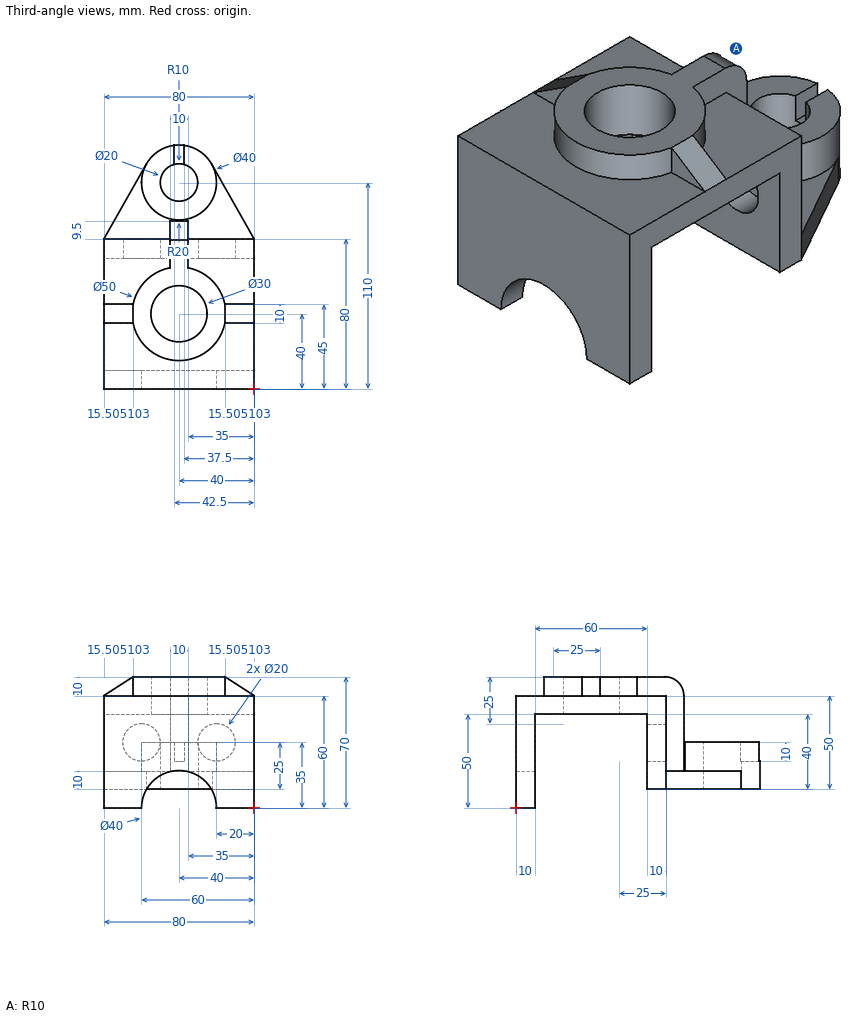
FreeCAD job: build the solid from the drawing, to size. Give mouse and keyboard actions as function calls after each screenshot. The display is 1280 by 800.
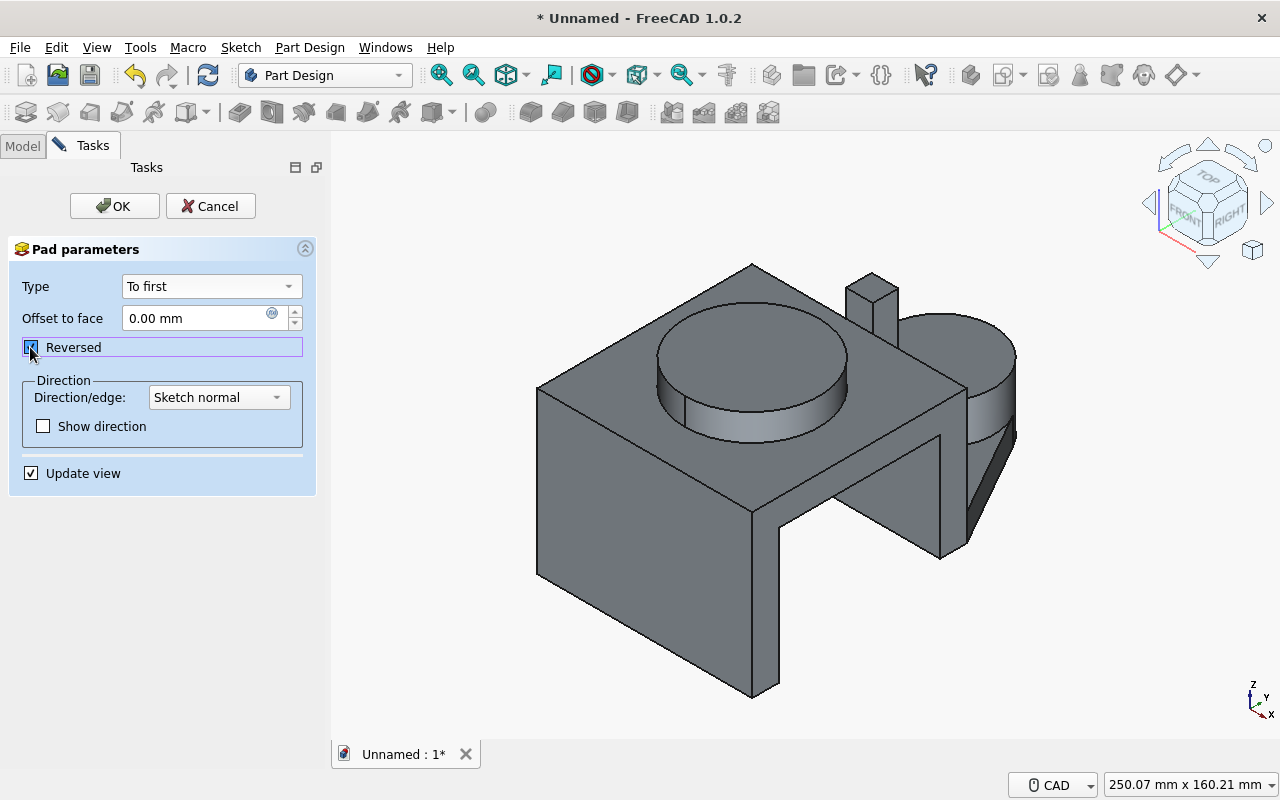
click(115, 206)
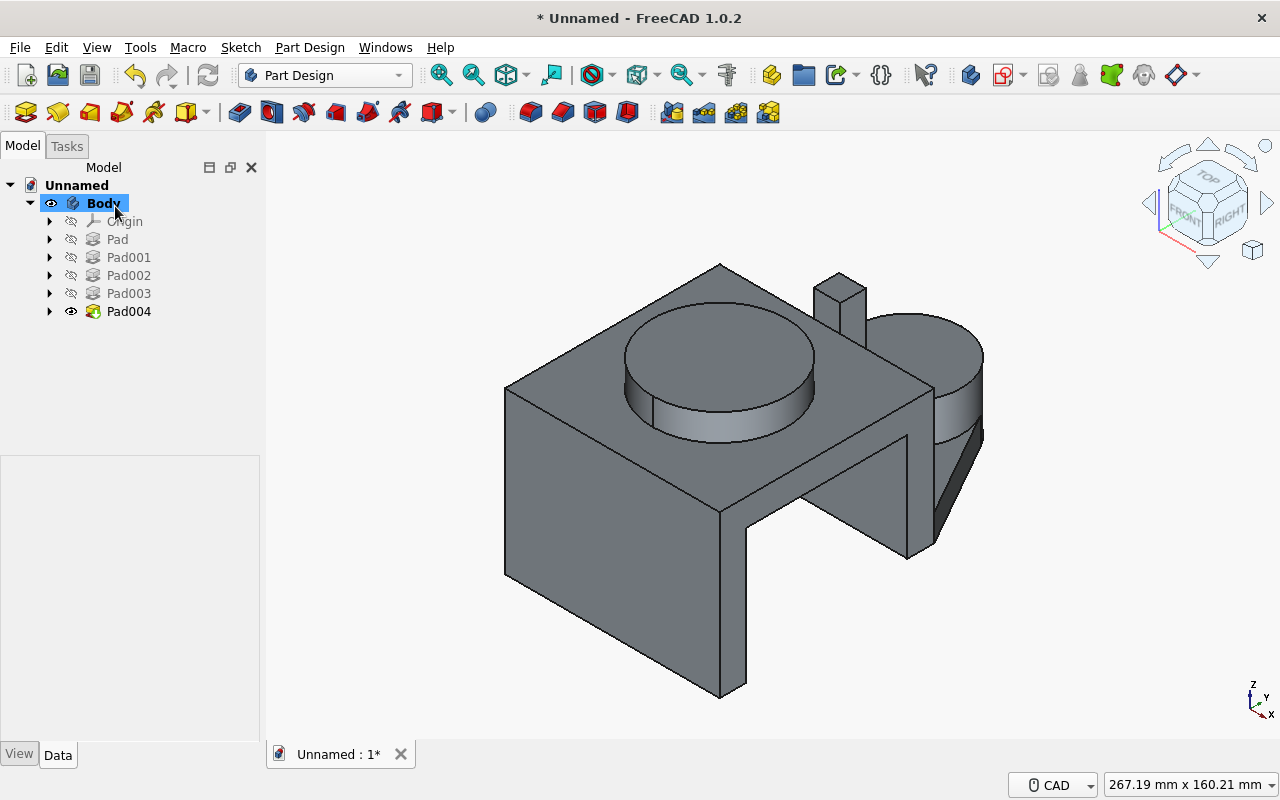
key(4)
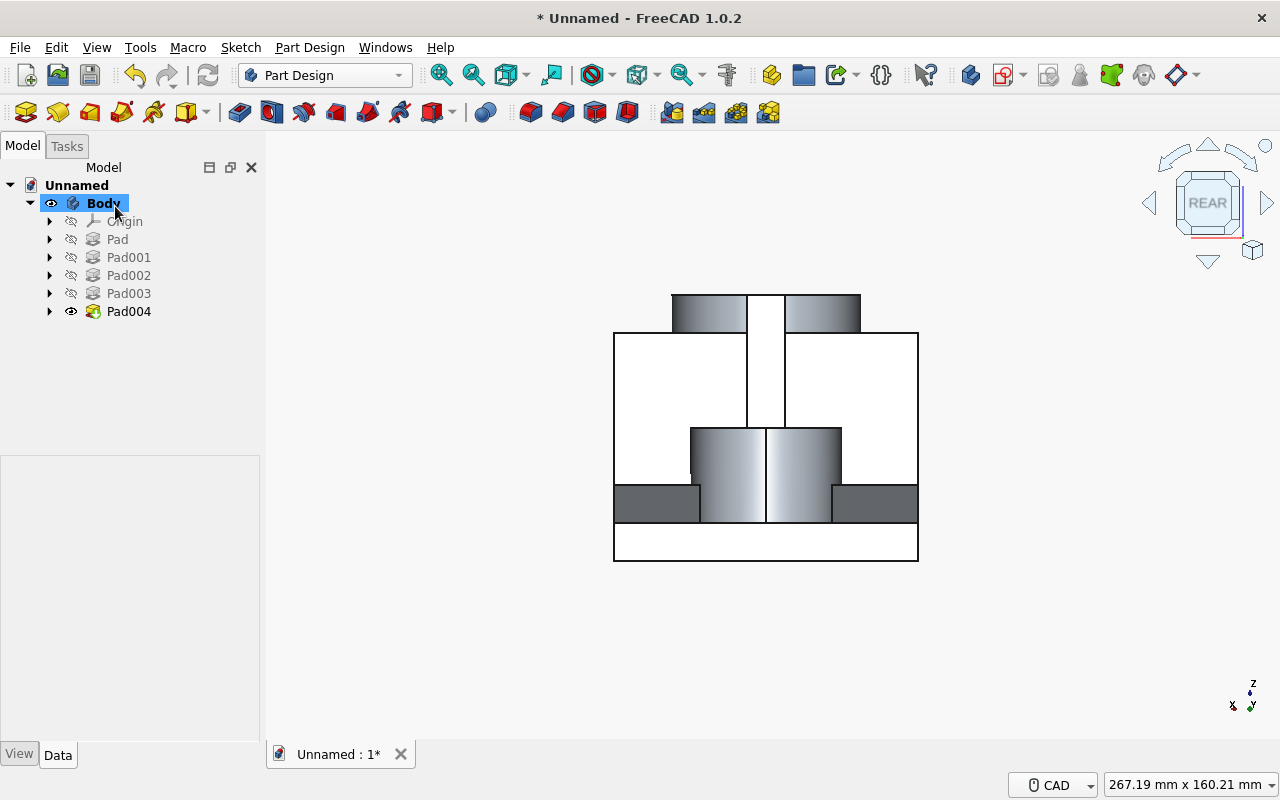
click(442, 76)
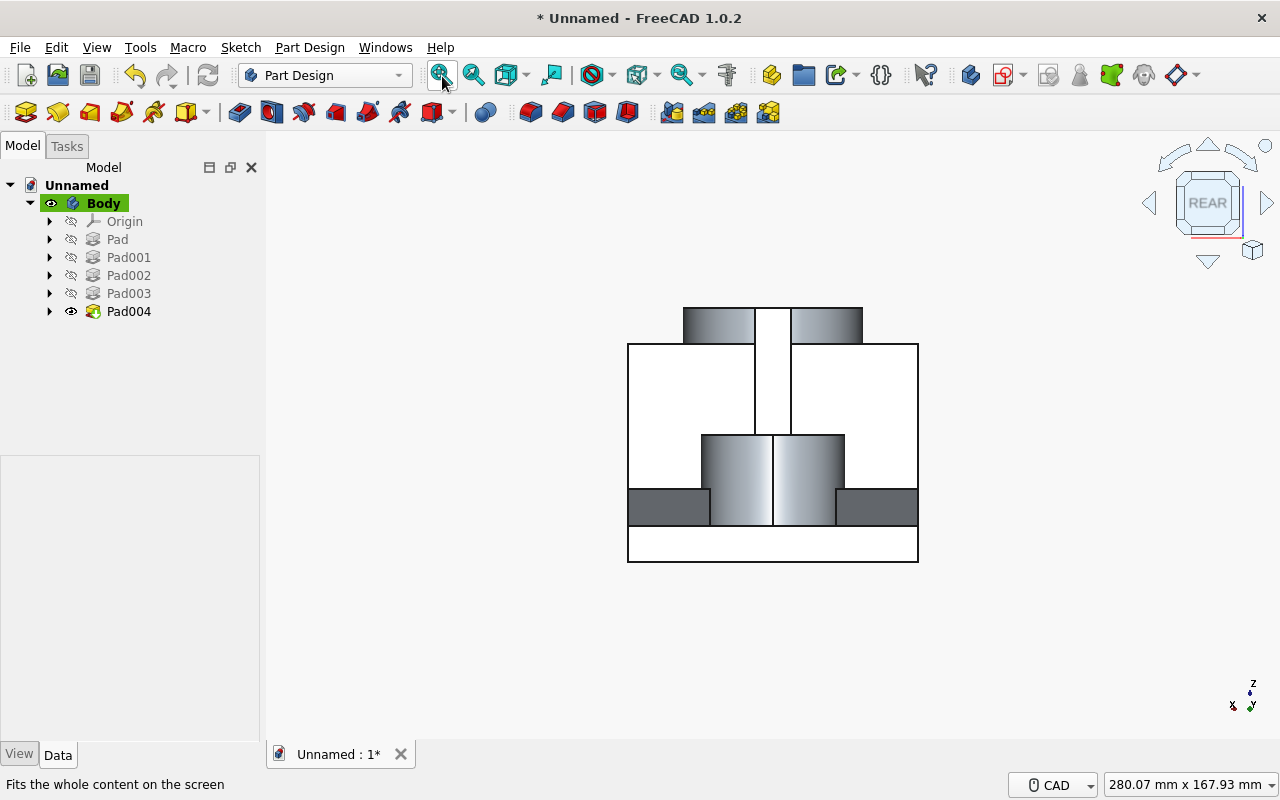
click(692, 416)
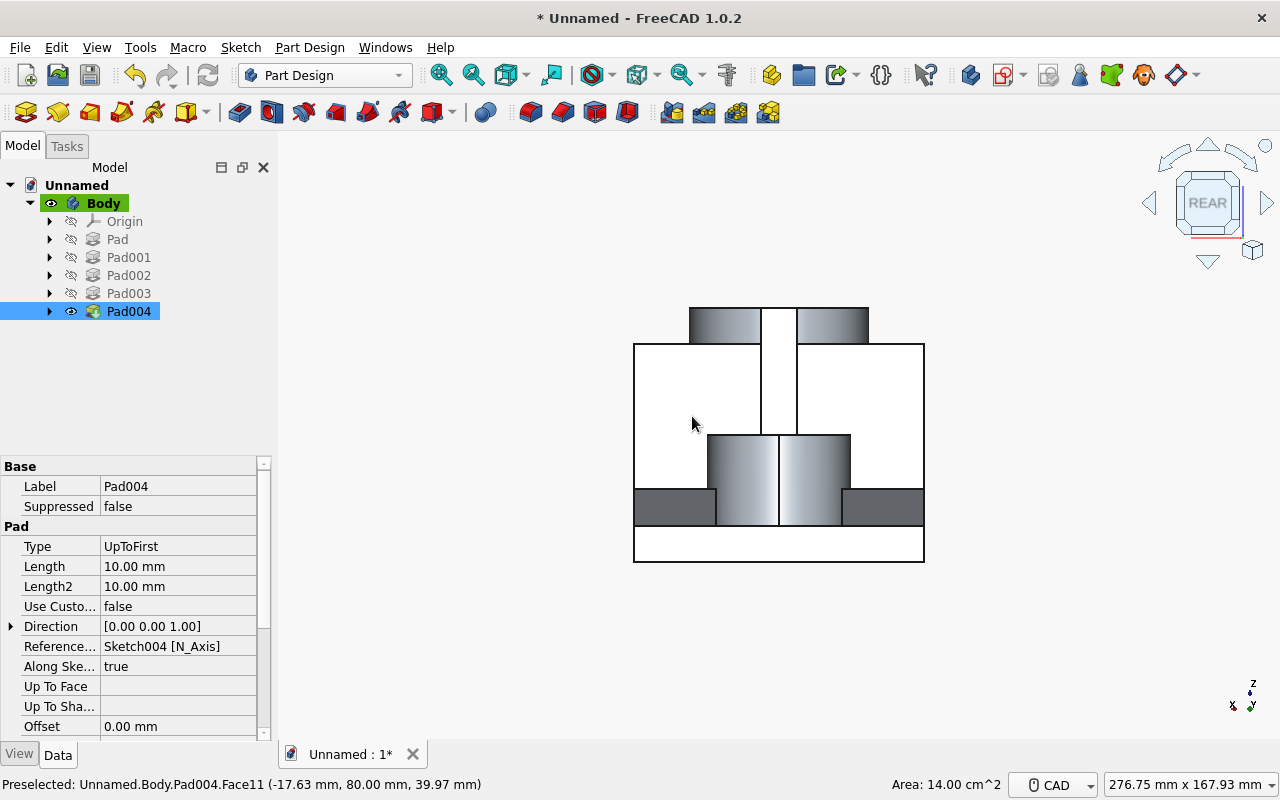
click(1004, 76)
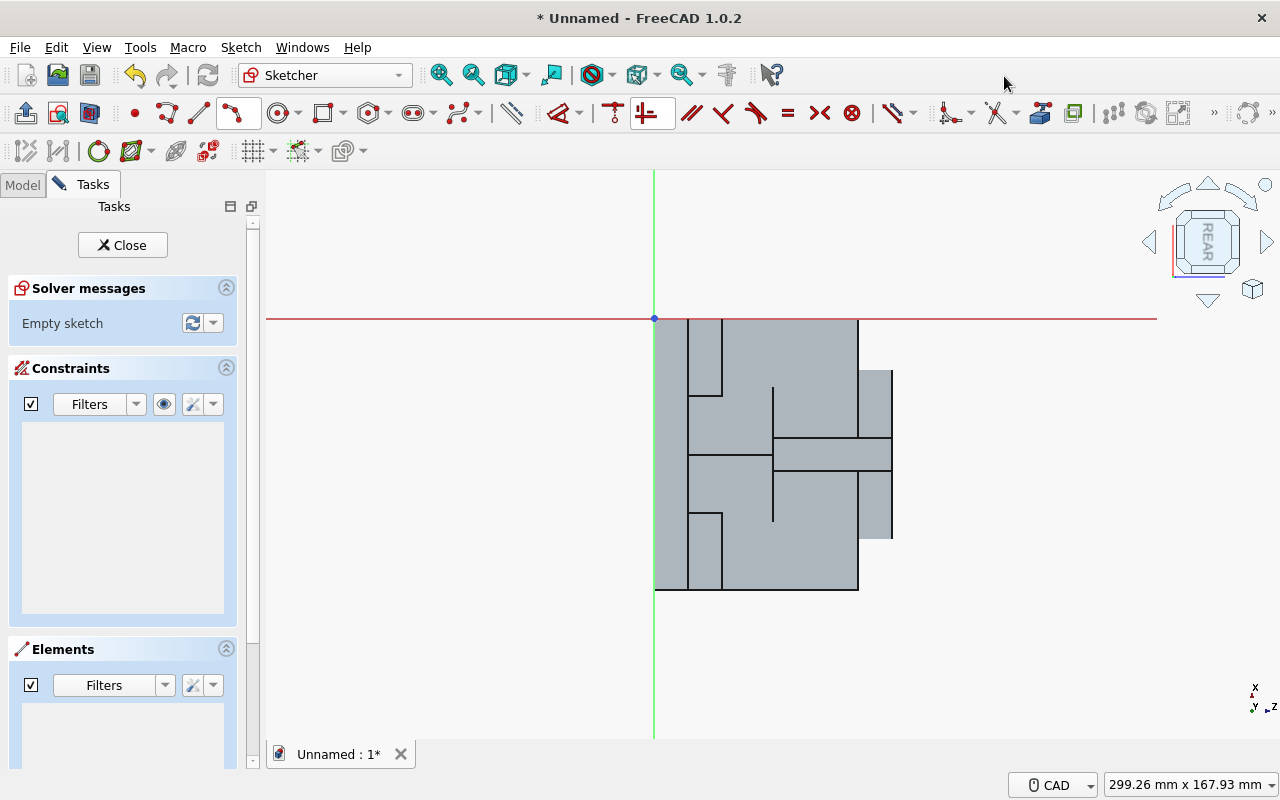
scroll(892, 455, up, 12)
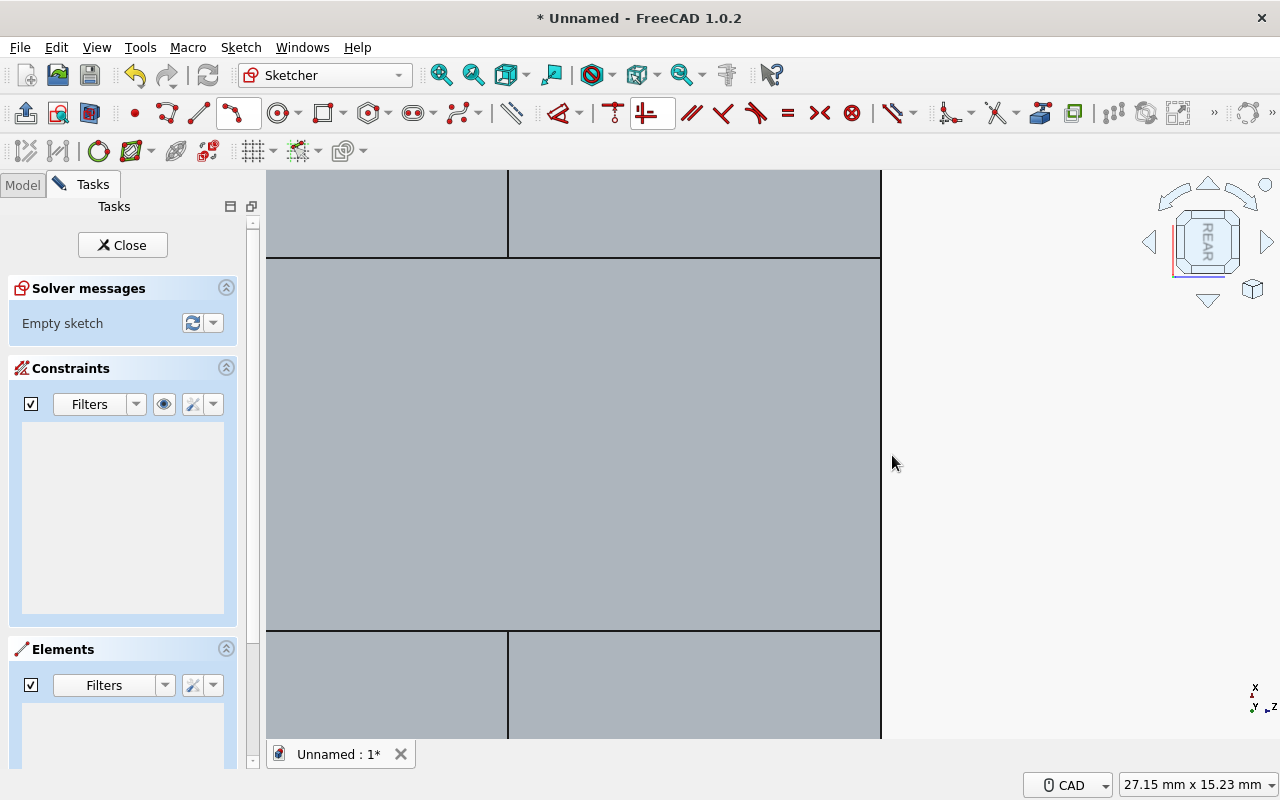
click(324, 114)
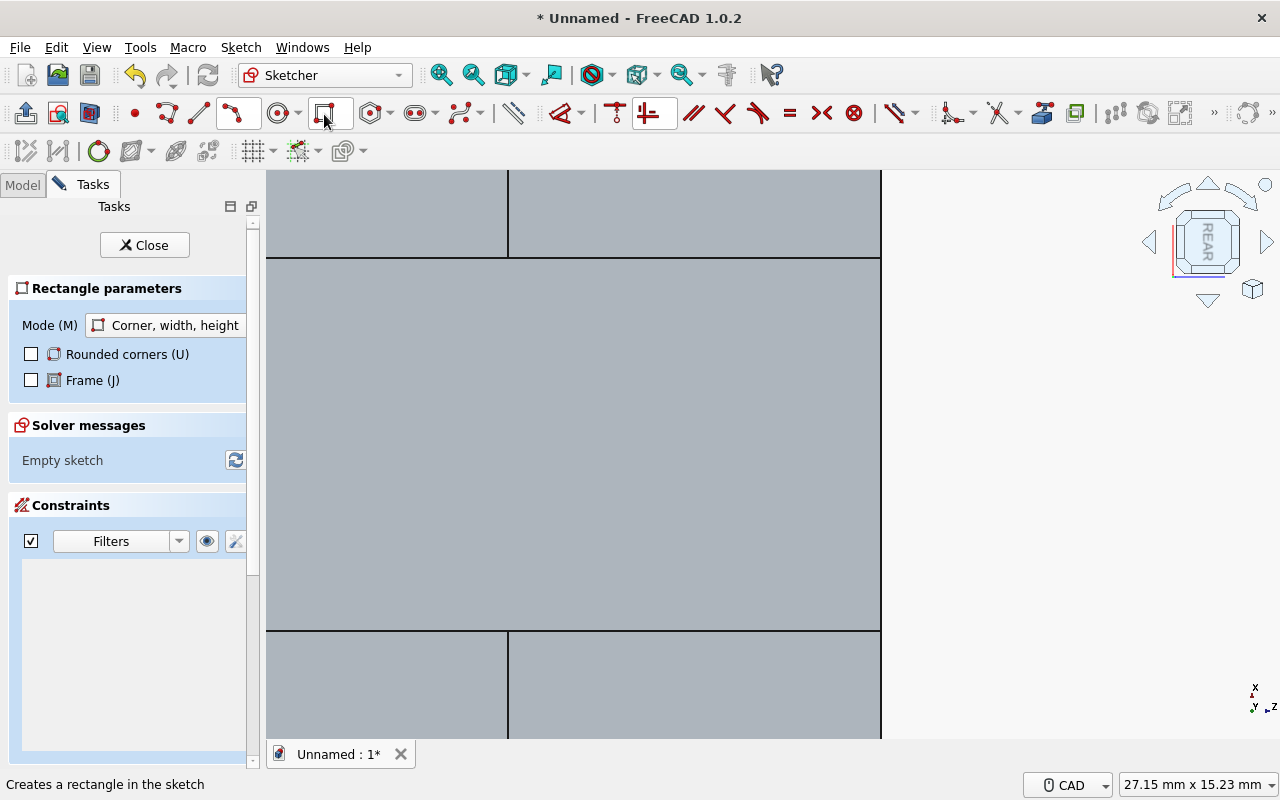
click(508, 258)
move(881, 631)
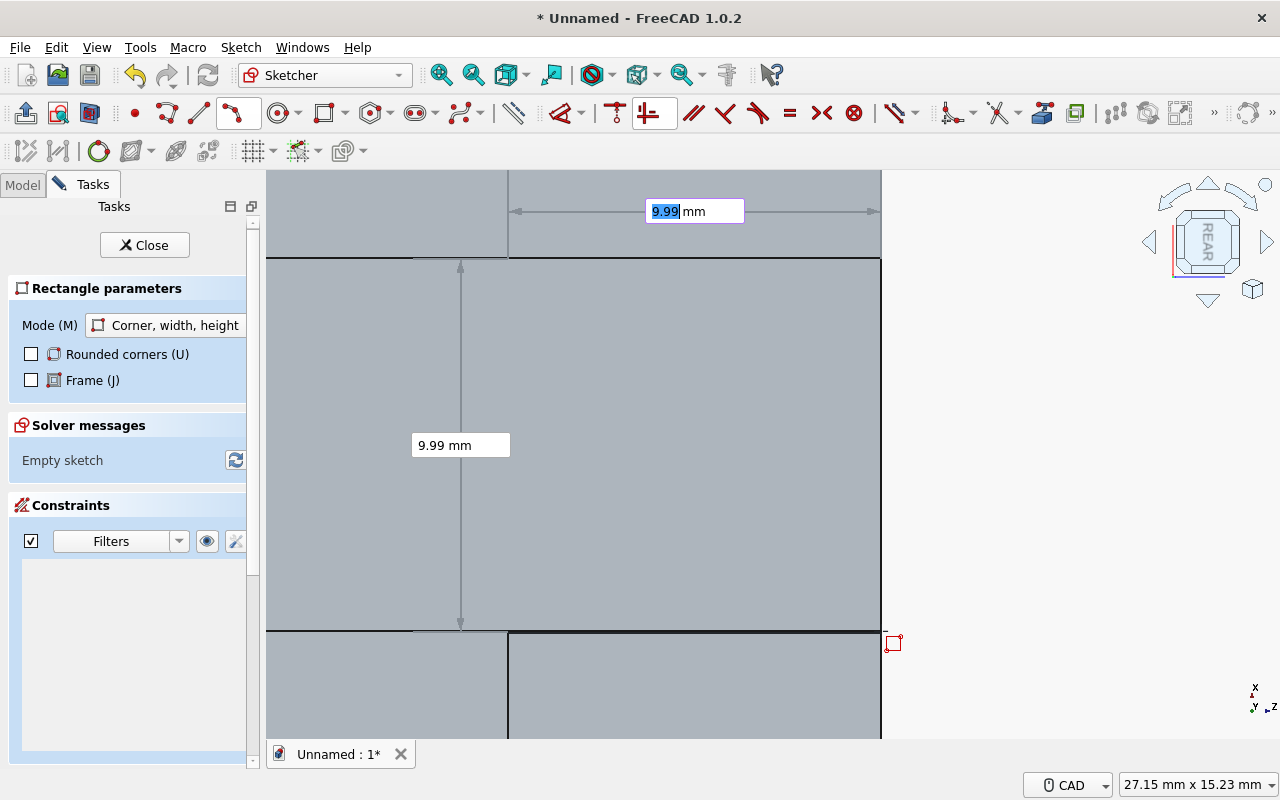
text(10)
key(Tab)
text(10)
key(Return)
key(Escape)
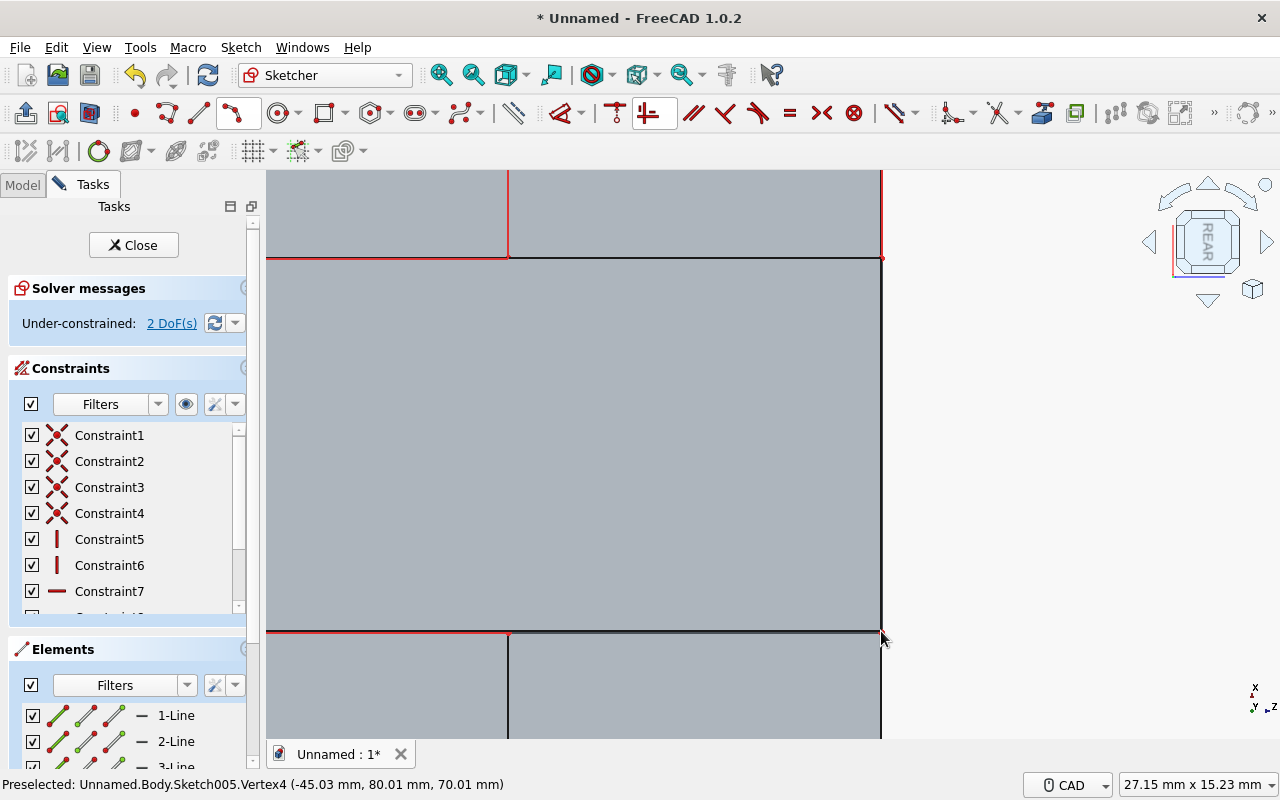
click(560, 114)